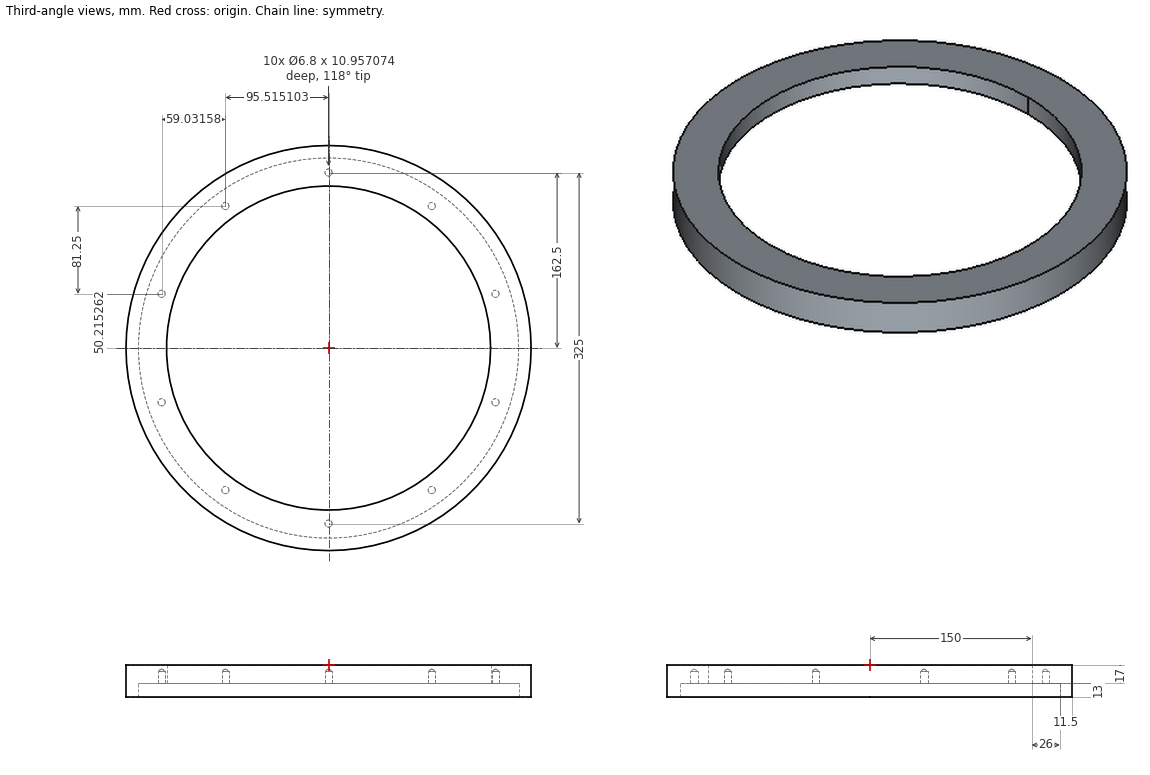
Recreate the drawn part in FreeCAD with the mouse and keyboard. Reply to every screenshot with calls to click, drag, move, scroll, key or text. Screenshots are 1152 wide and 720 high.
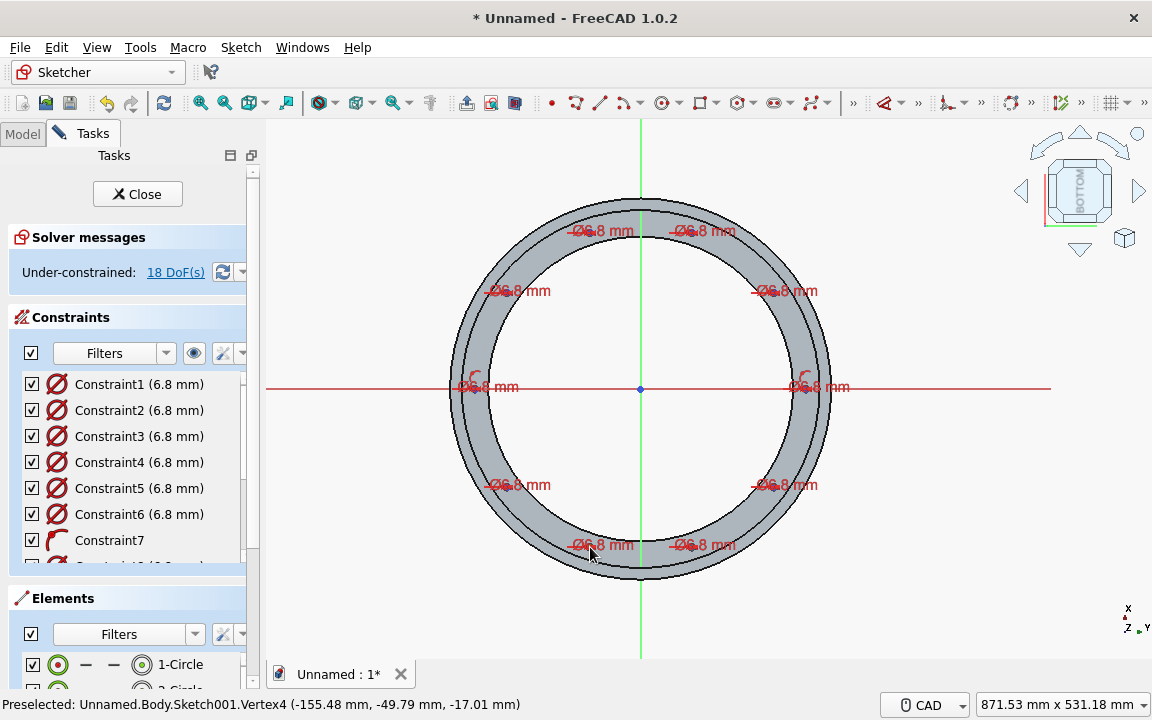
click(641, 596)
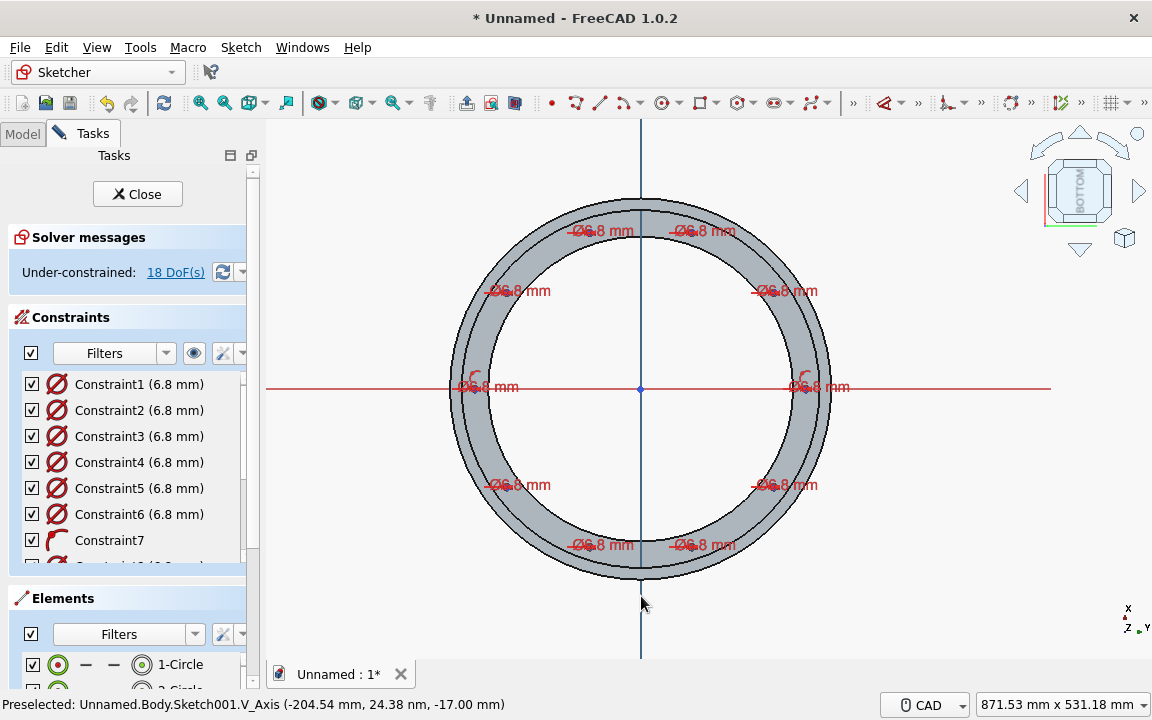
key(s)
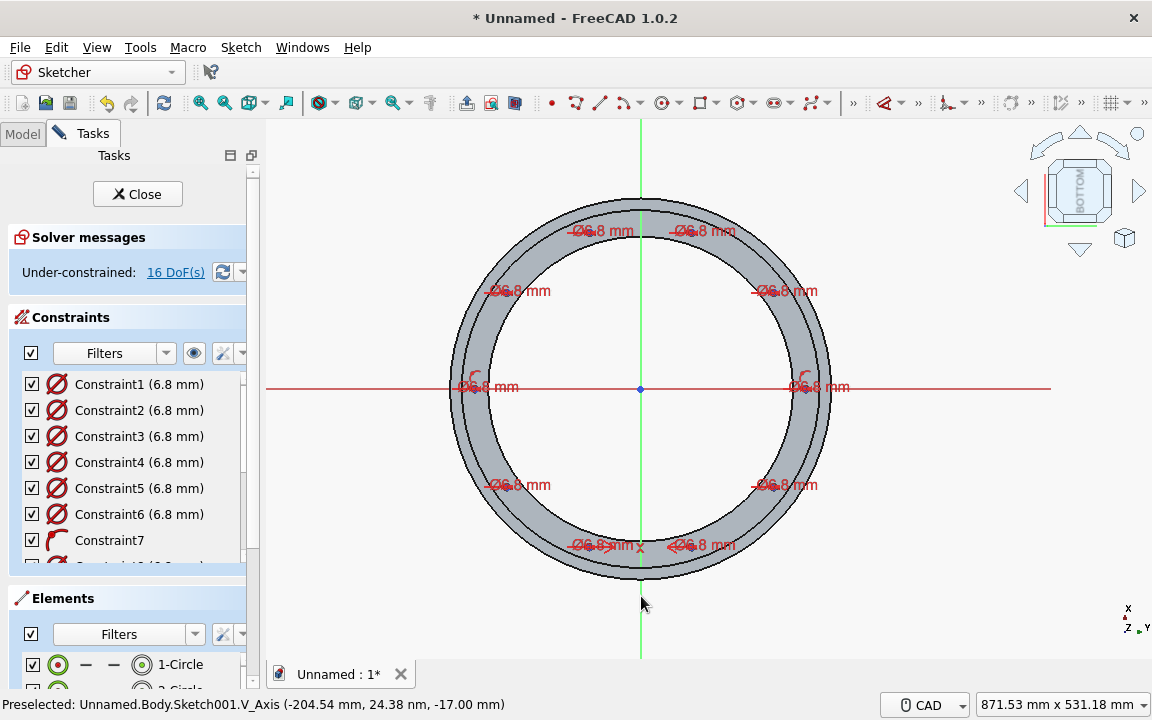
click(774, 487)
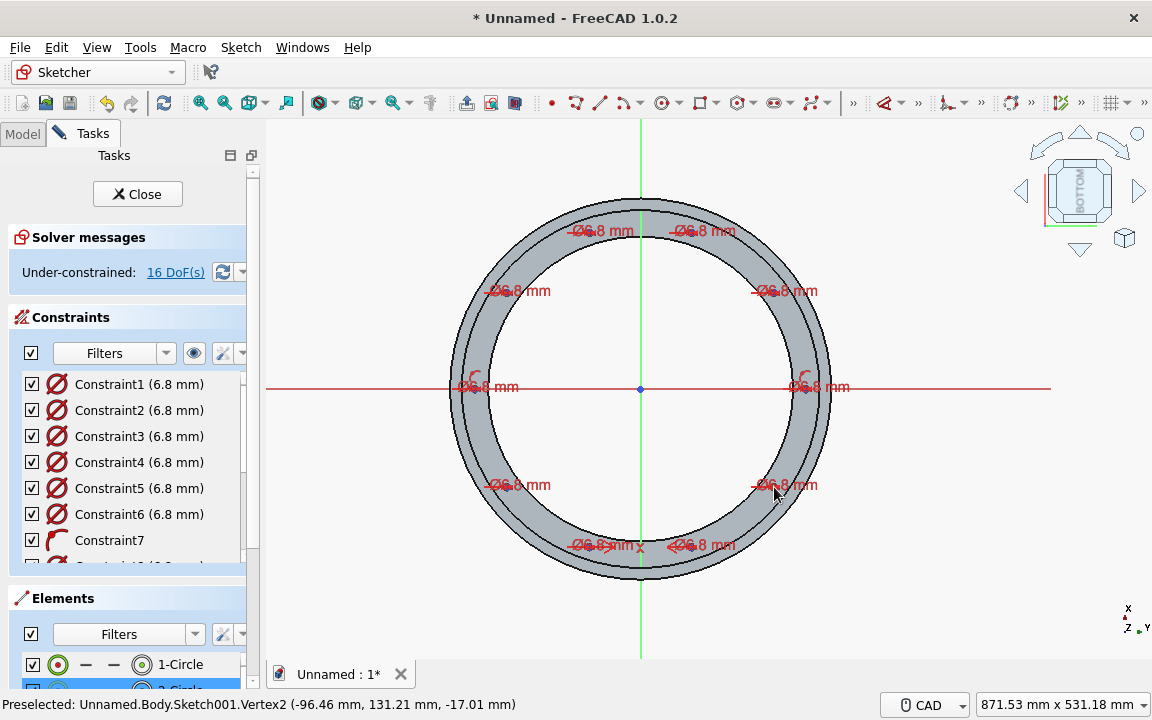
click(507, 487)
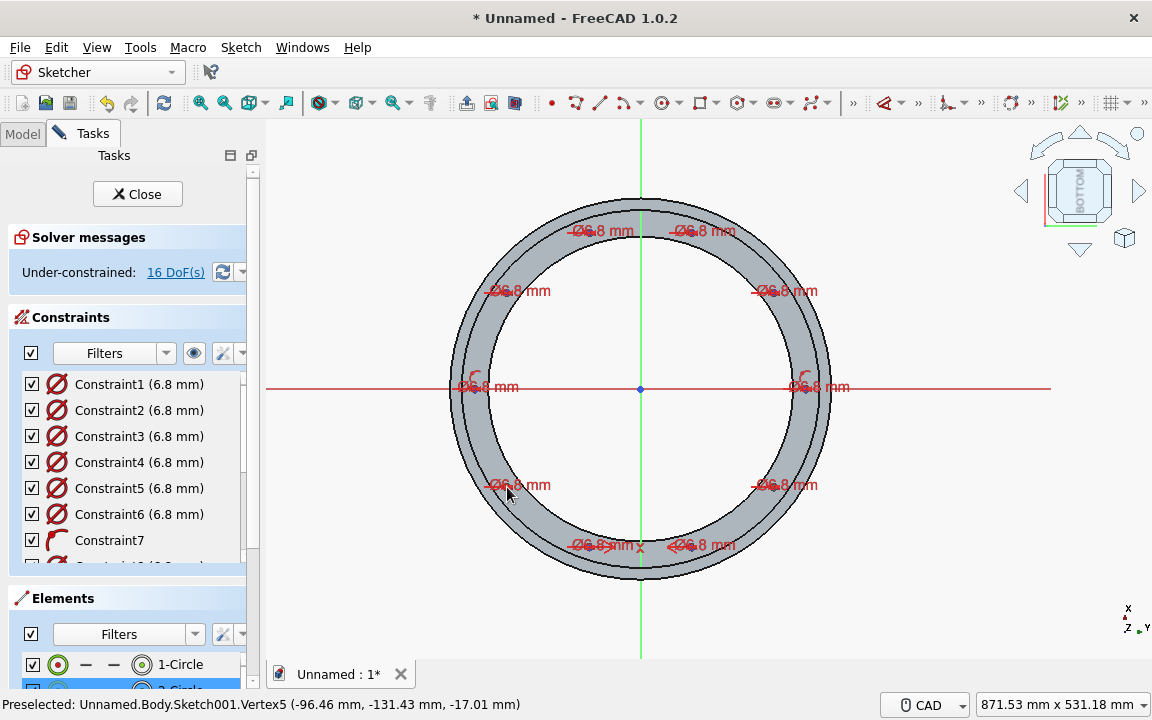
click(641, 596)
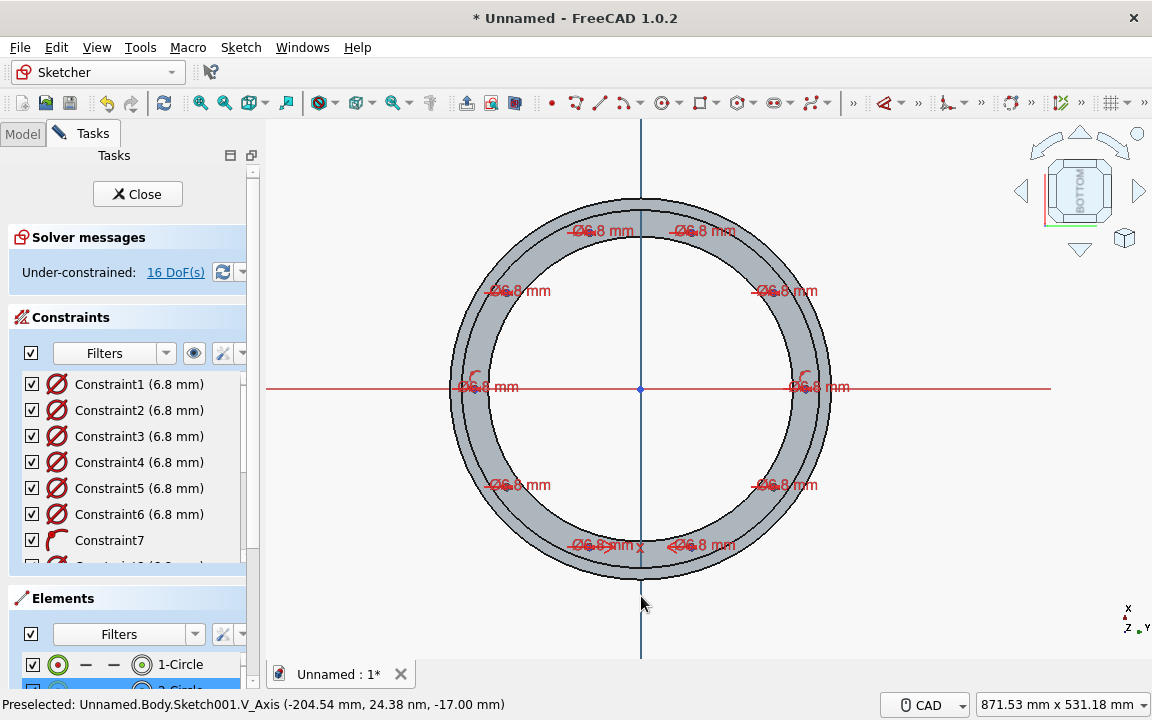
key(s)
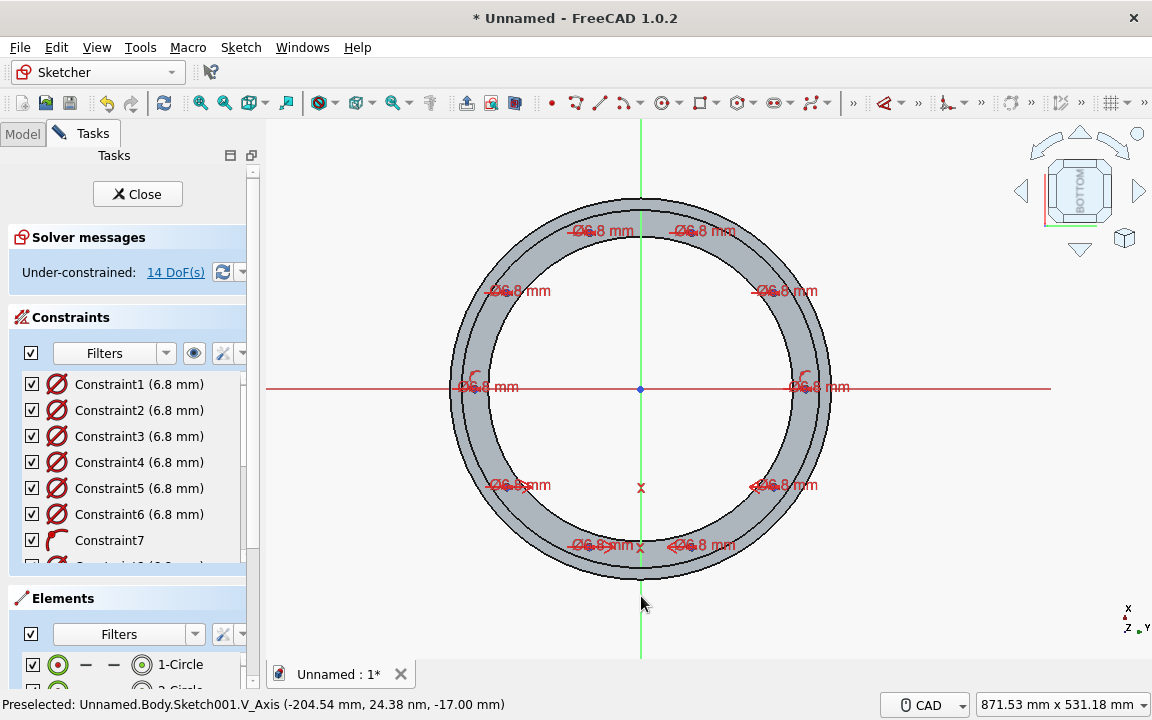
click(507, 487)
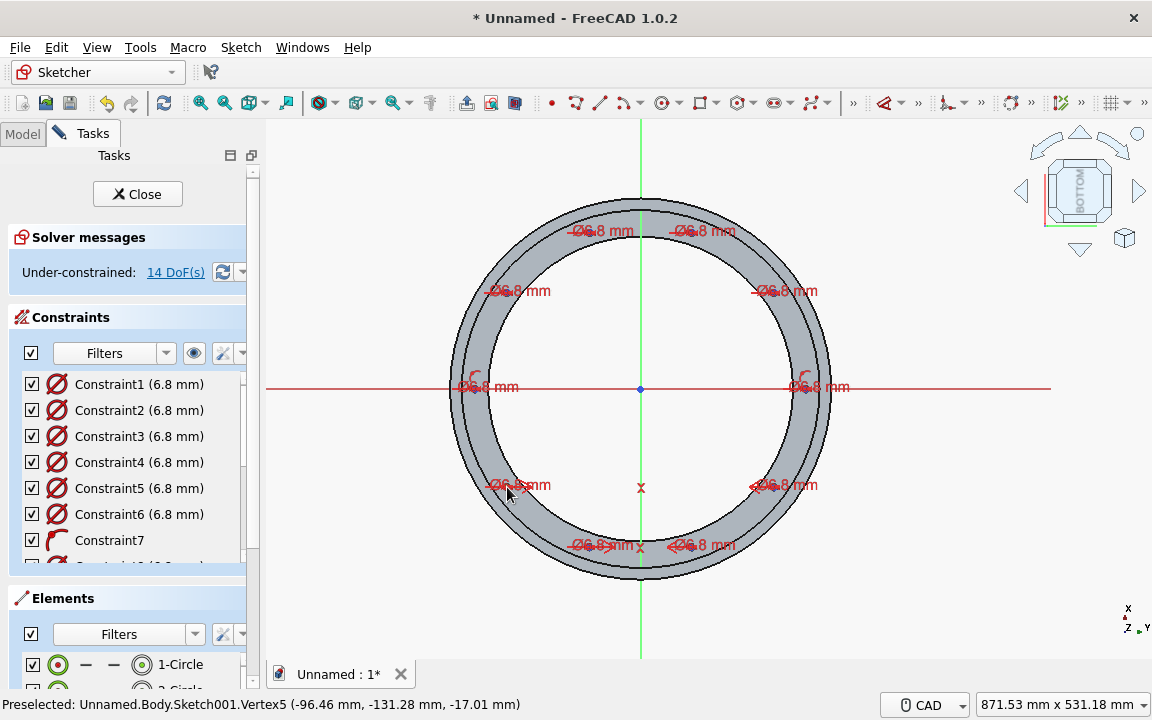
click(507, 293)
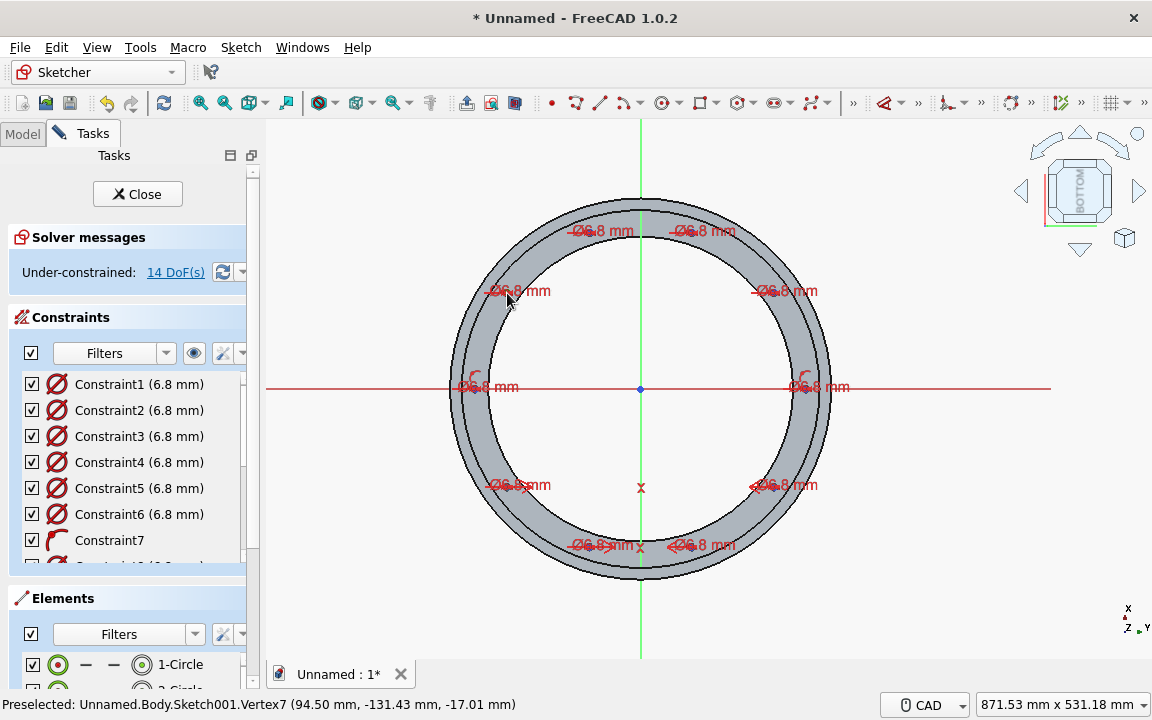
click(344, 389)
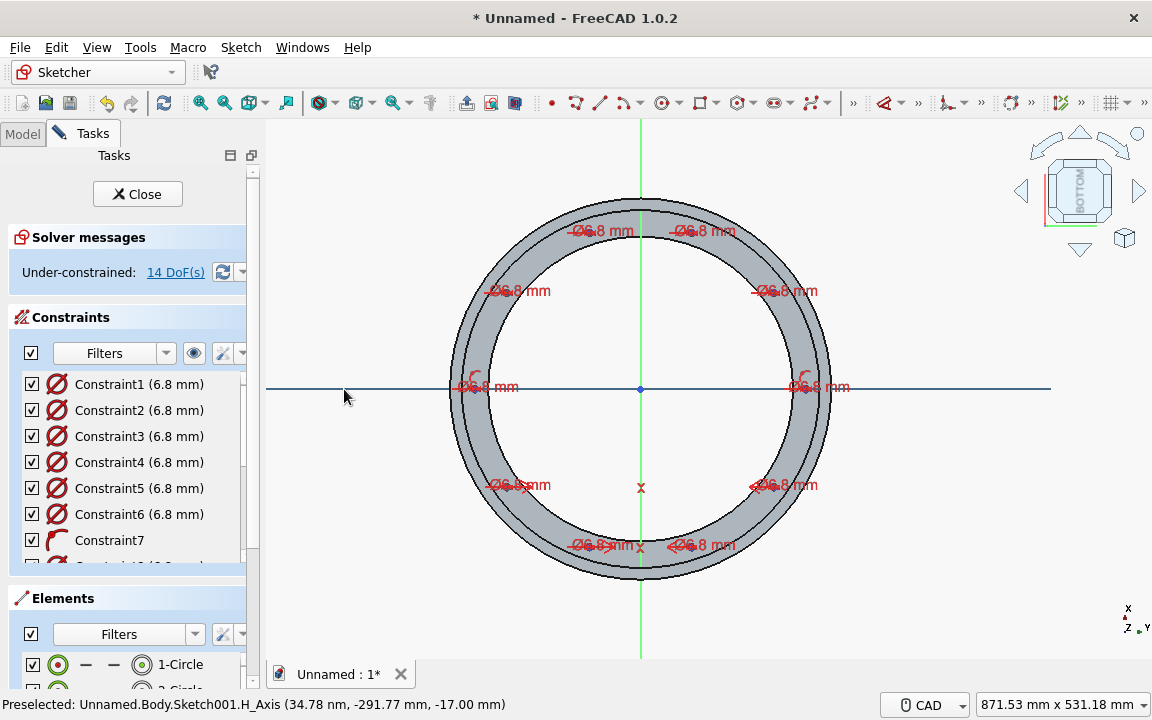
key(s)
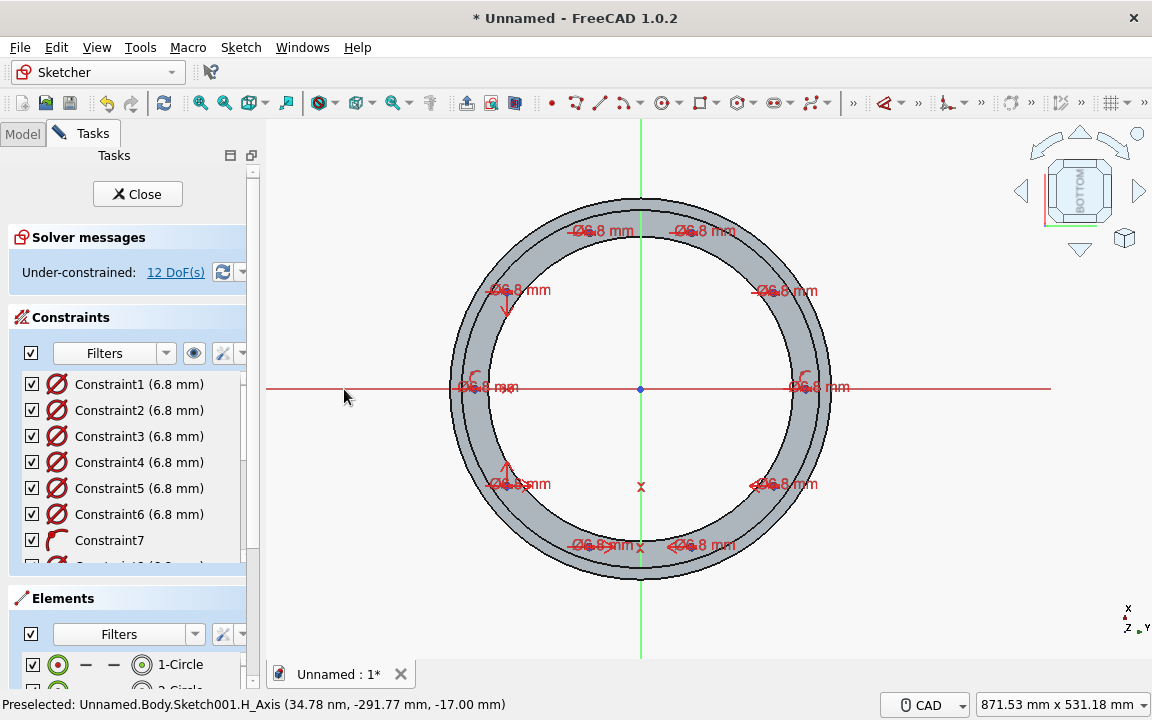
click(590, 547)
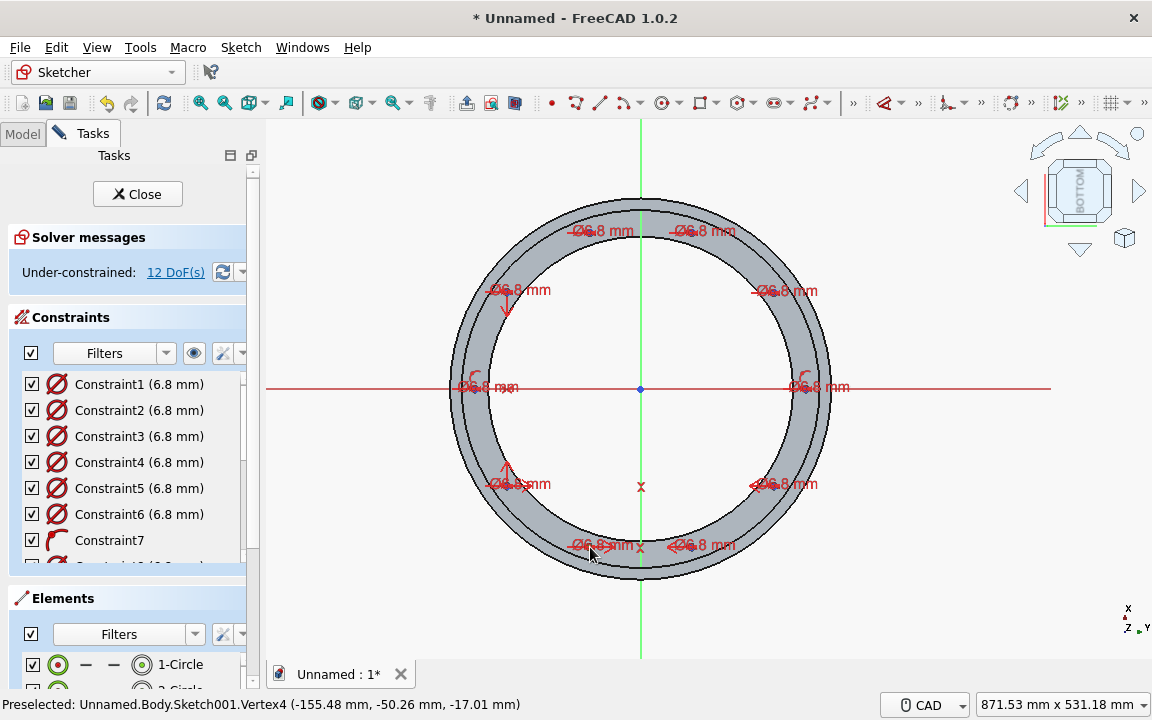
click(590, 233)